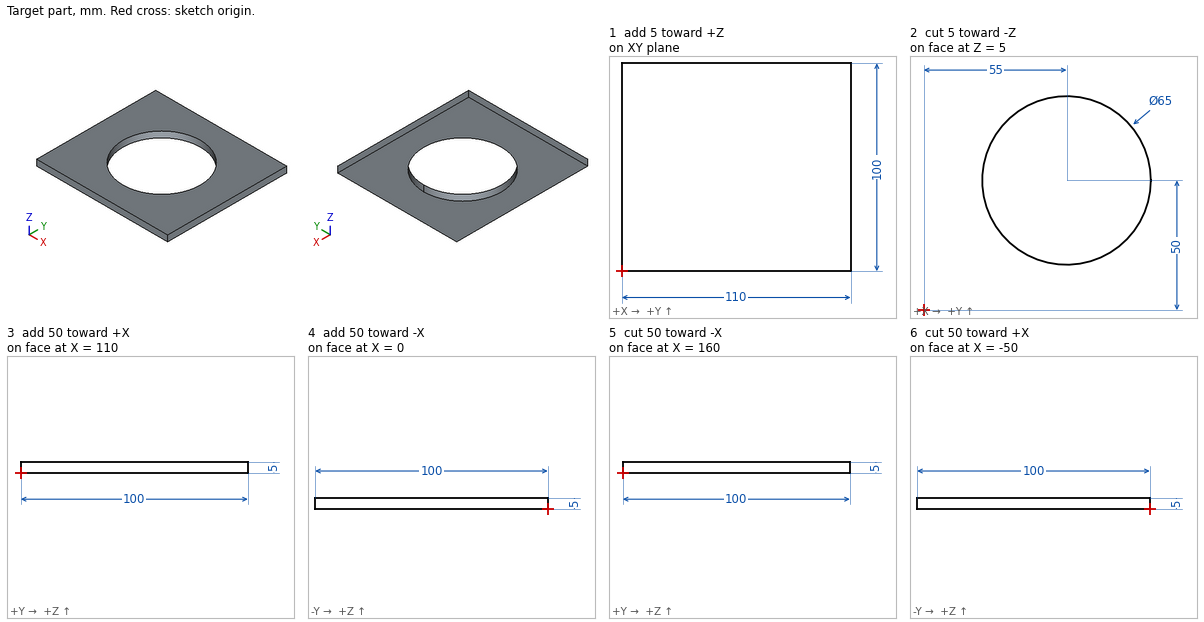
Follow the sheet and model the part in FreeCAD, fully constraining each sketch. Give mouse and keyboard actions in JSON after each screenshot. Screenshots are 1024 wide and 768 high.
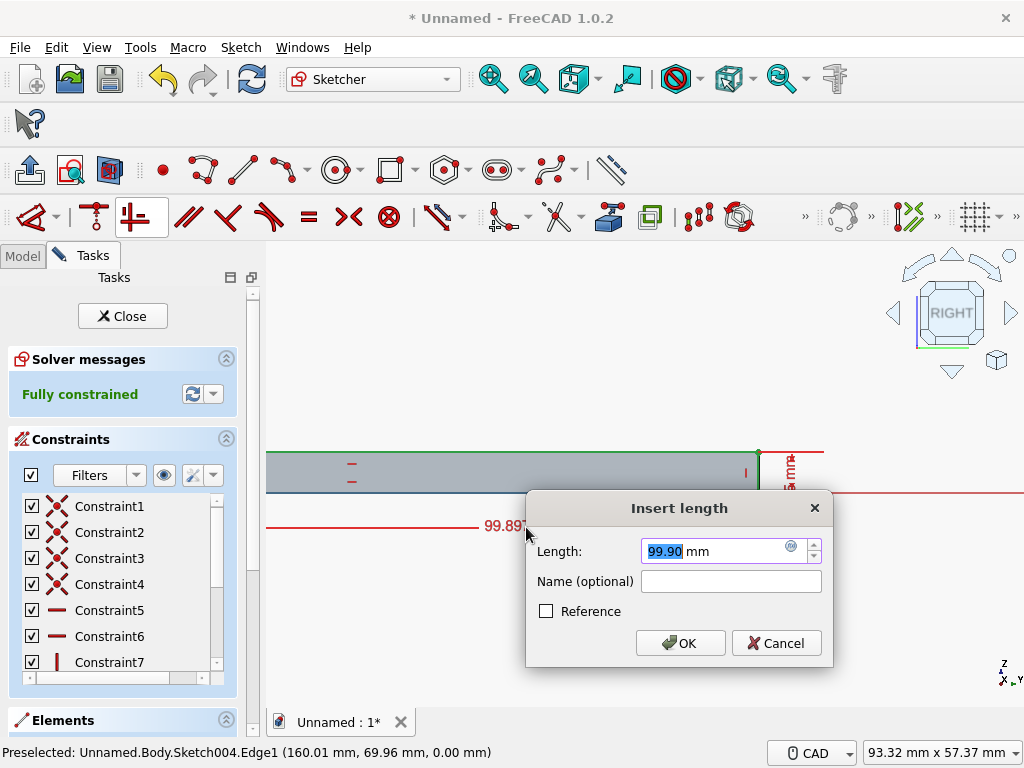
{"action": "type", "text": "100"}
{"action": "key", "text": "Return"}
{"action": "key", "text": "Escape"}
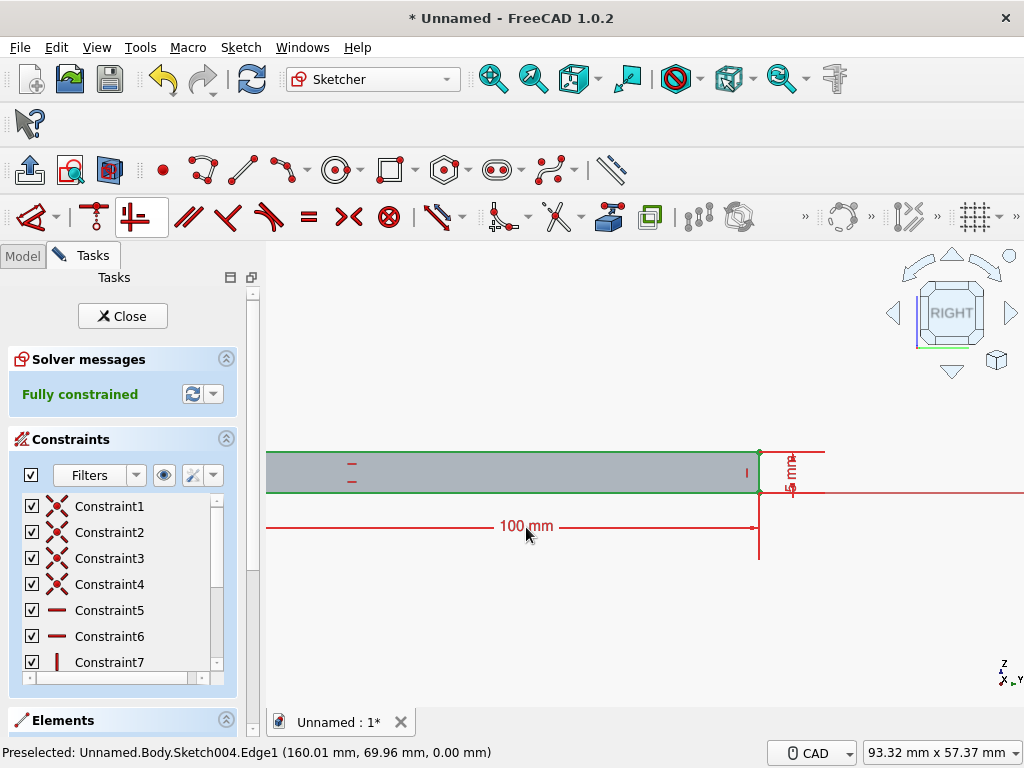
{"action": "left_click", "coordinate": [123, 316]}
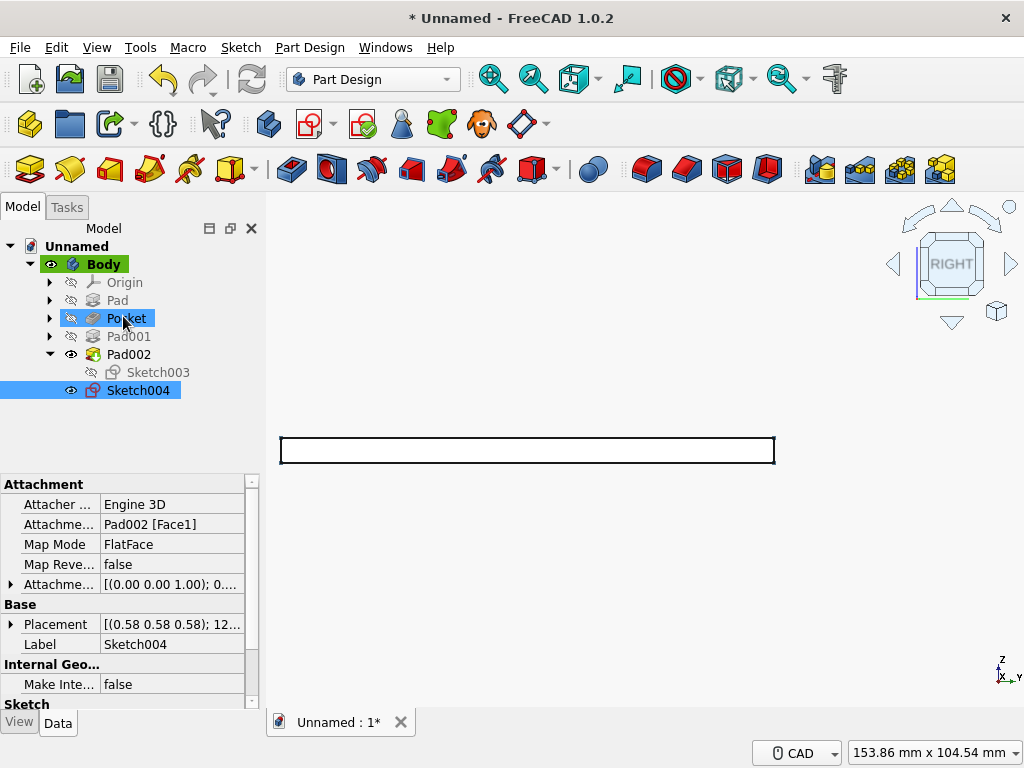
{"action": "left_click", "coordinate": [292, 170]}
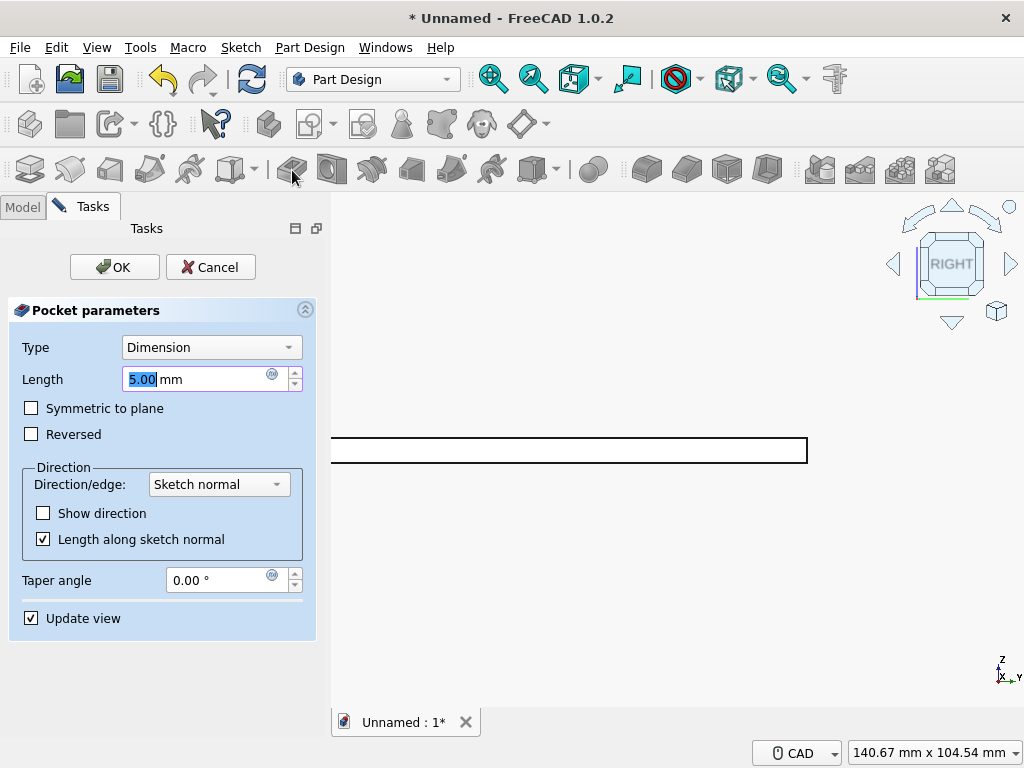
{"action": "type", "text": "50"}
{"action": "key", "text": "Tab"}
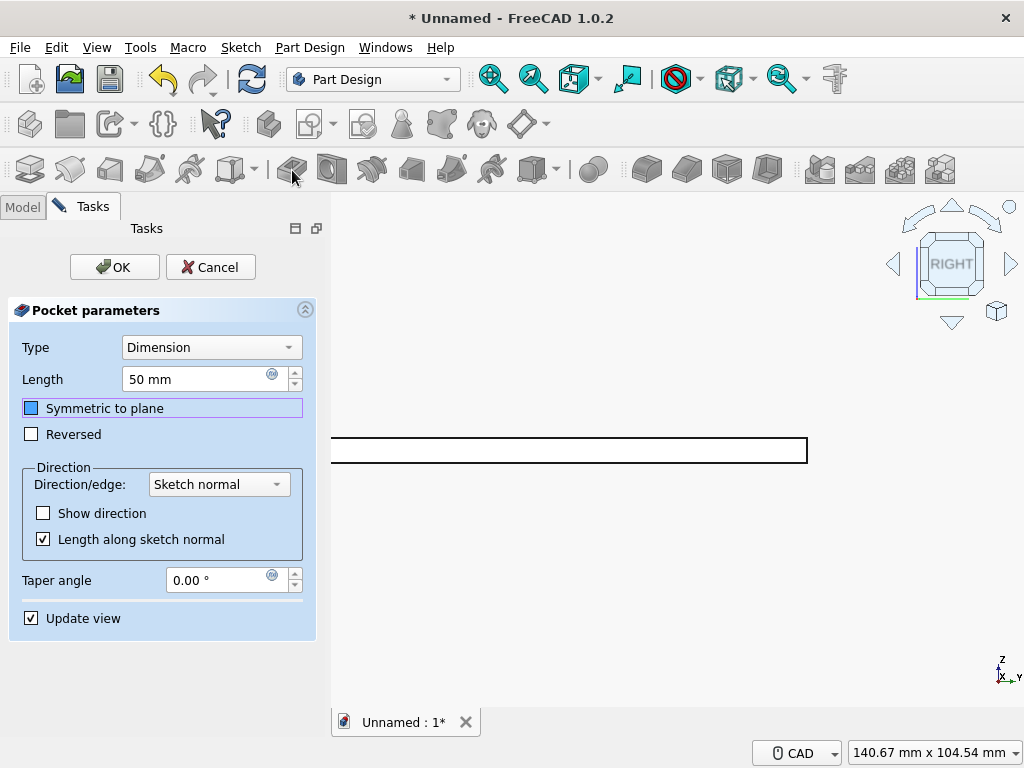
{"action": "left_click", "coordinate": [115, 267]}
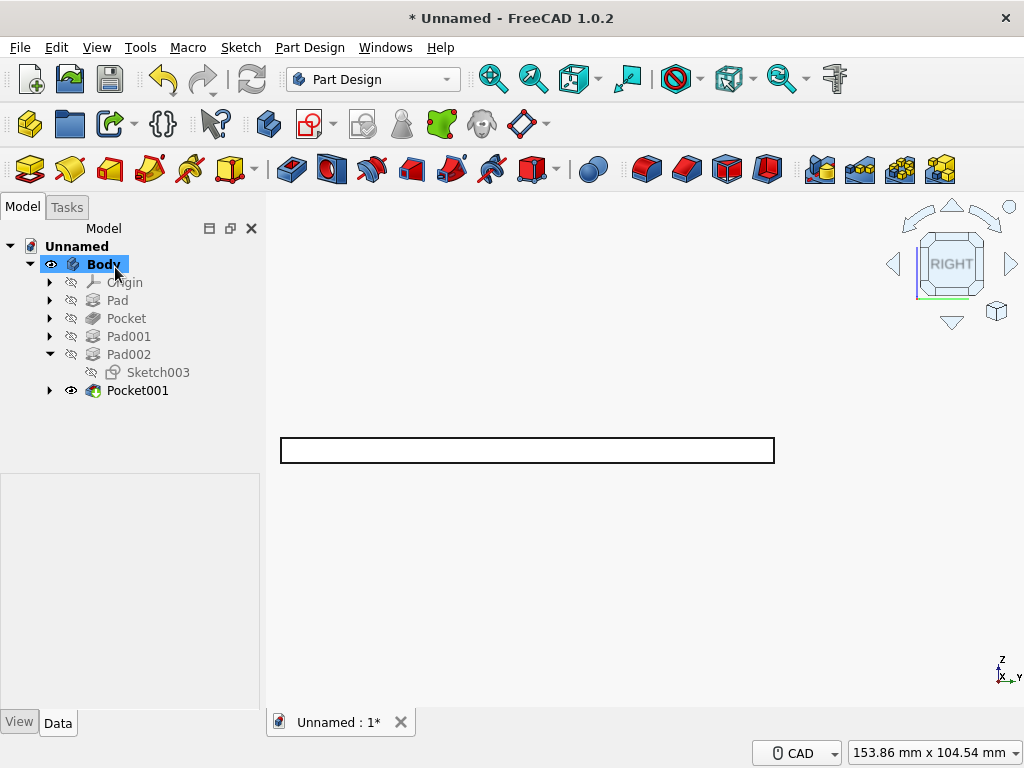
{"action": "key", "text": "6"}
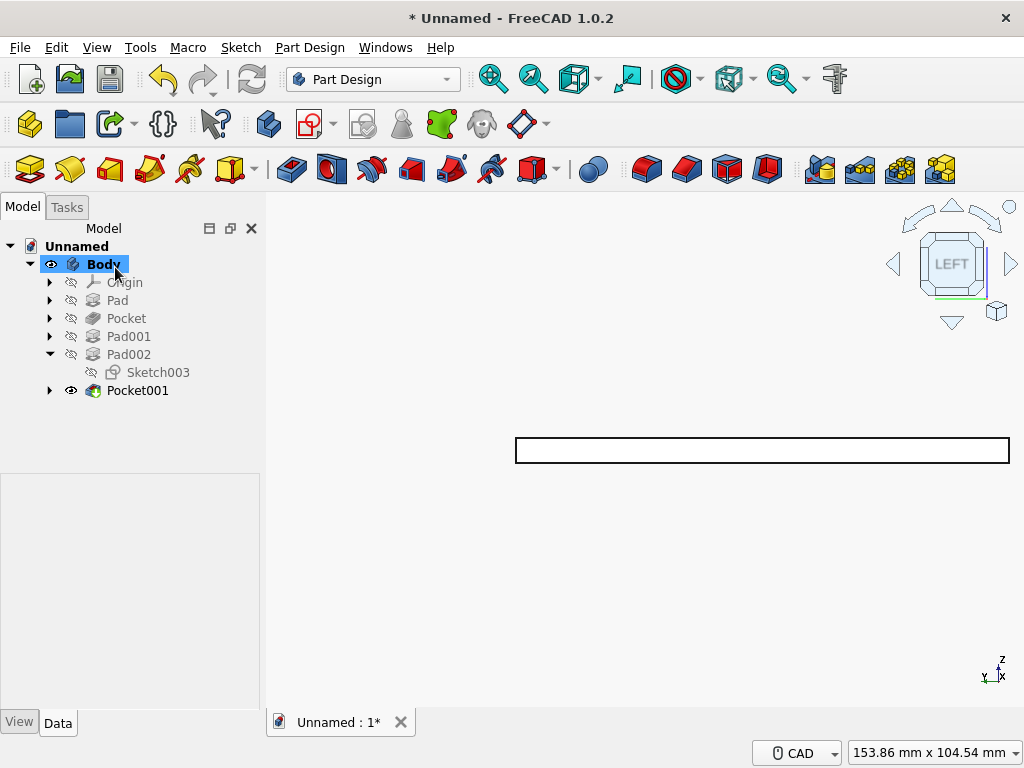
{"action": "left_click", "coordinate": [551, 450]}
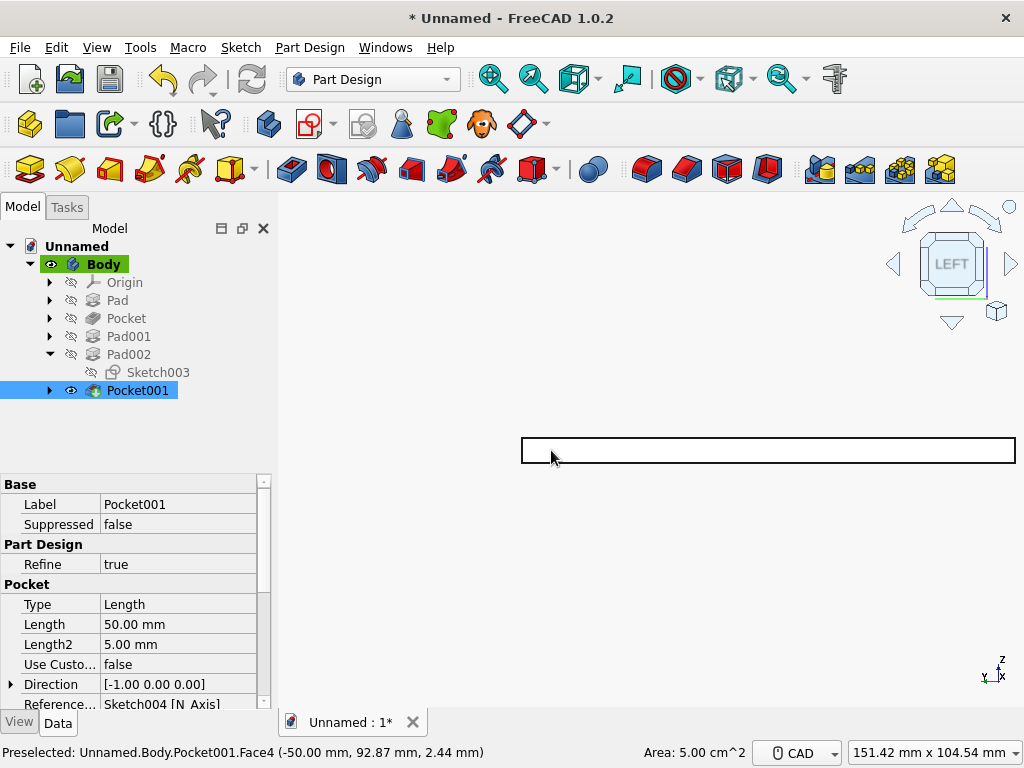
{"action": "left_click", "coordinate": [310, 124]}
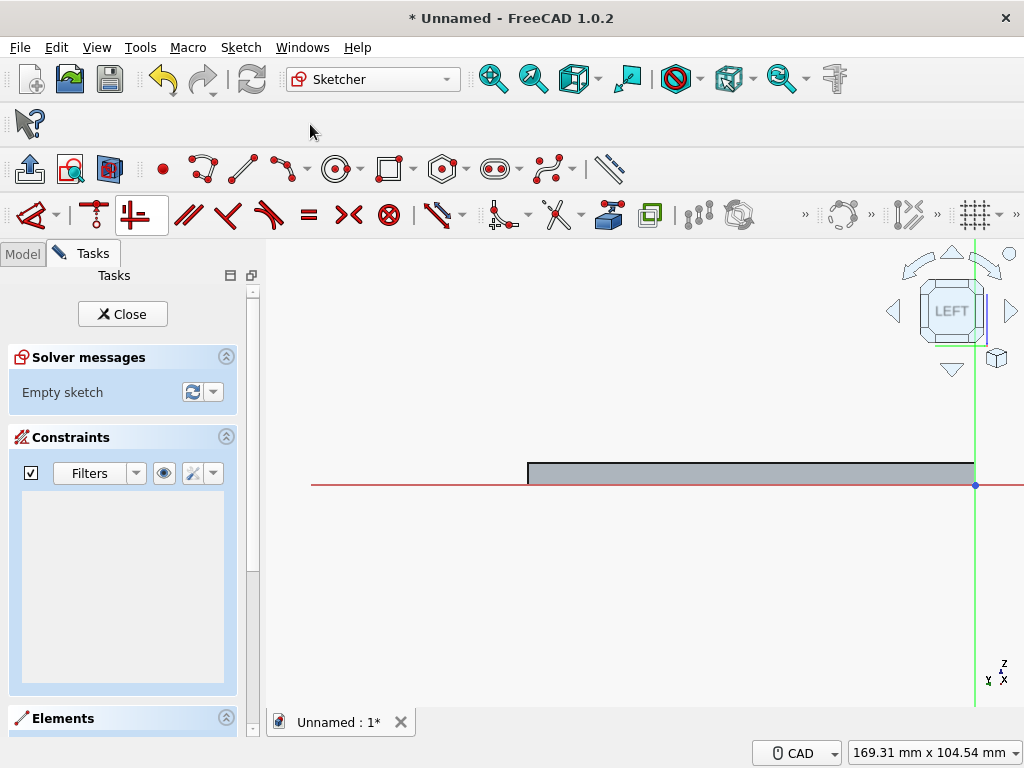
{"action": "scroll", "coordinate": [294, 471], "scroll_direction": "down", "scroll_amount": 2}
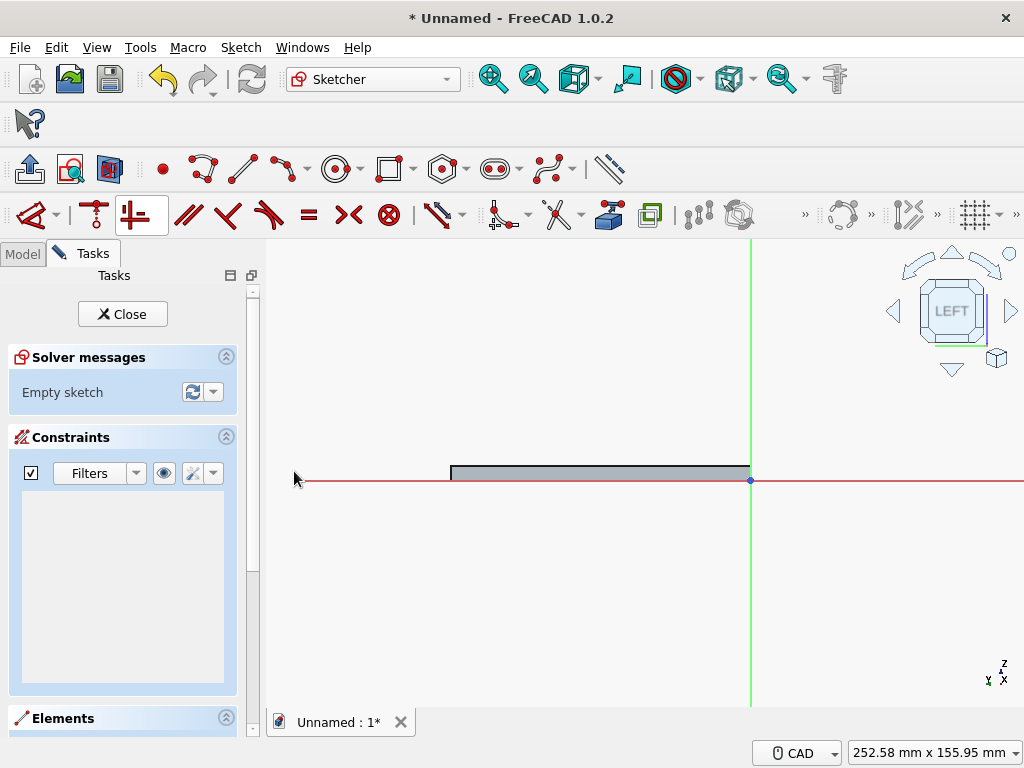
{"action": "left_click", "coordinate": [390, 170]}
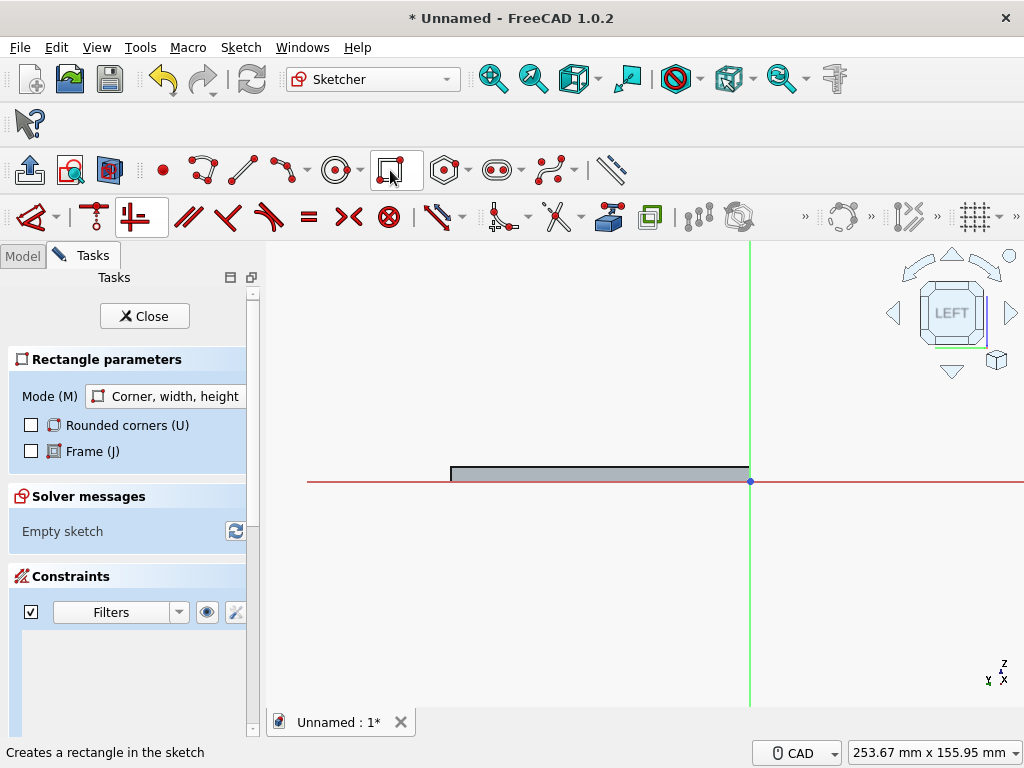
{"action": "left_click", "coordinate": [750, 482]}
{"action": "left_click", "coordinate": [451, 467]}
{"action": "key", "text": "Escape"}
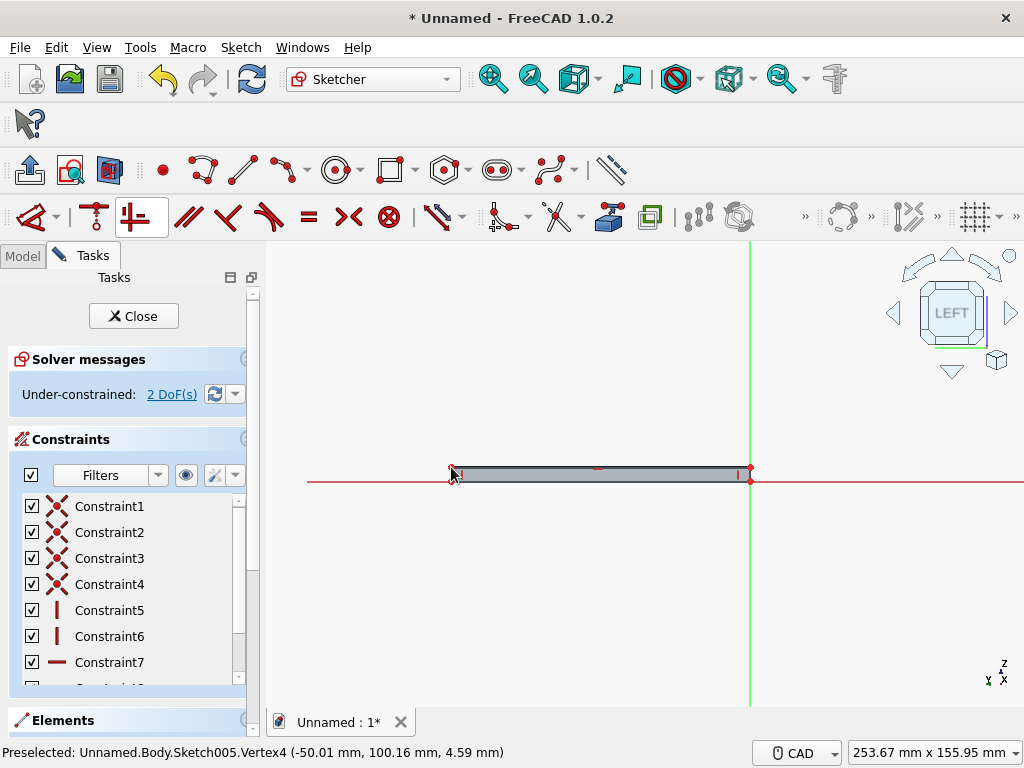
{"action": "left_click", "coordinate": [32, 218]}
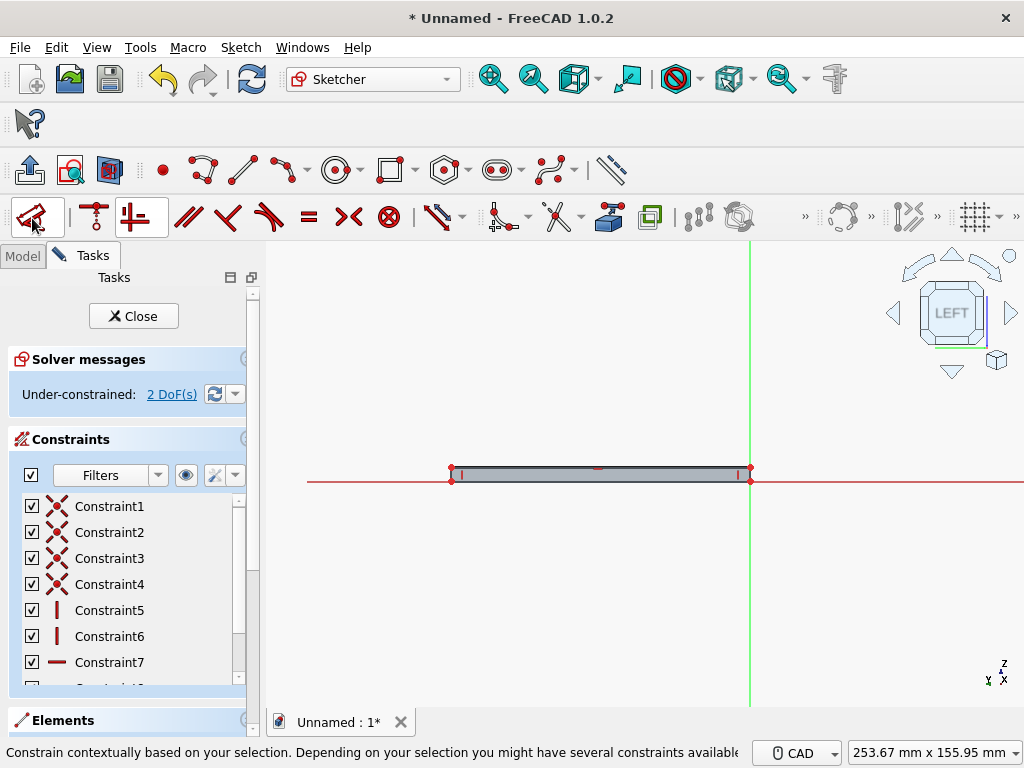
{"action": "scroll", "coordinate": [750, 475], "scroll_direction": "up", "scroll_amount": 5}